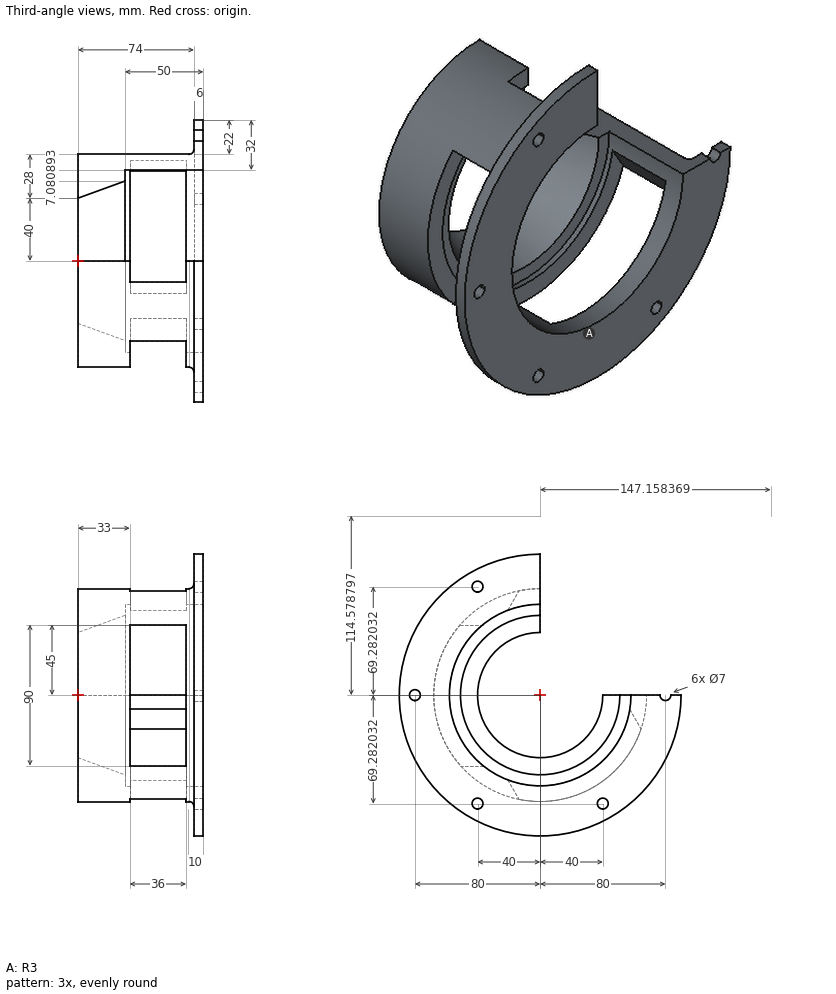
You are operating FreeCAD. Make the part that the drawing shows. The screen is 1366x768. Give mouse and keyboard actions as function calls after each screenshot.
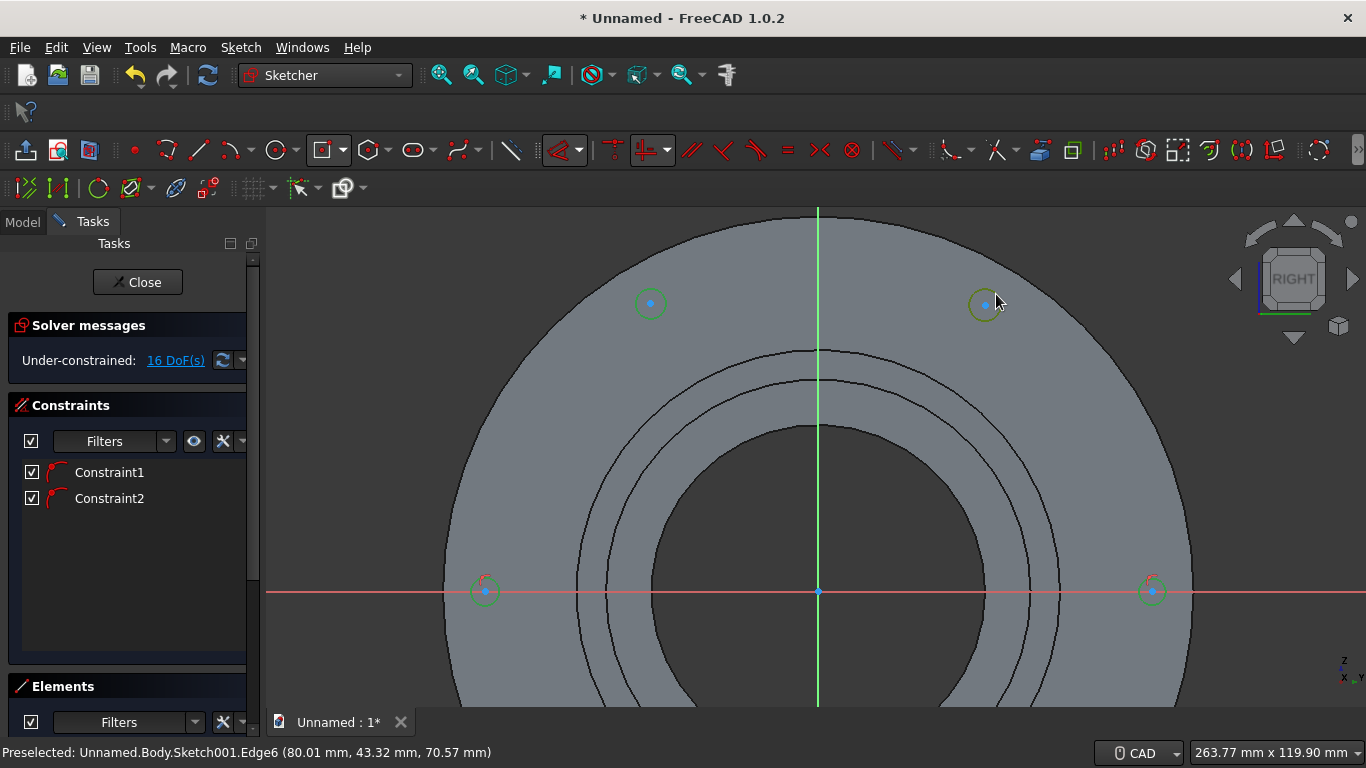
click(788, 150)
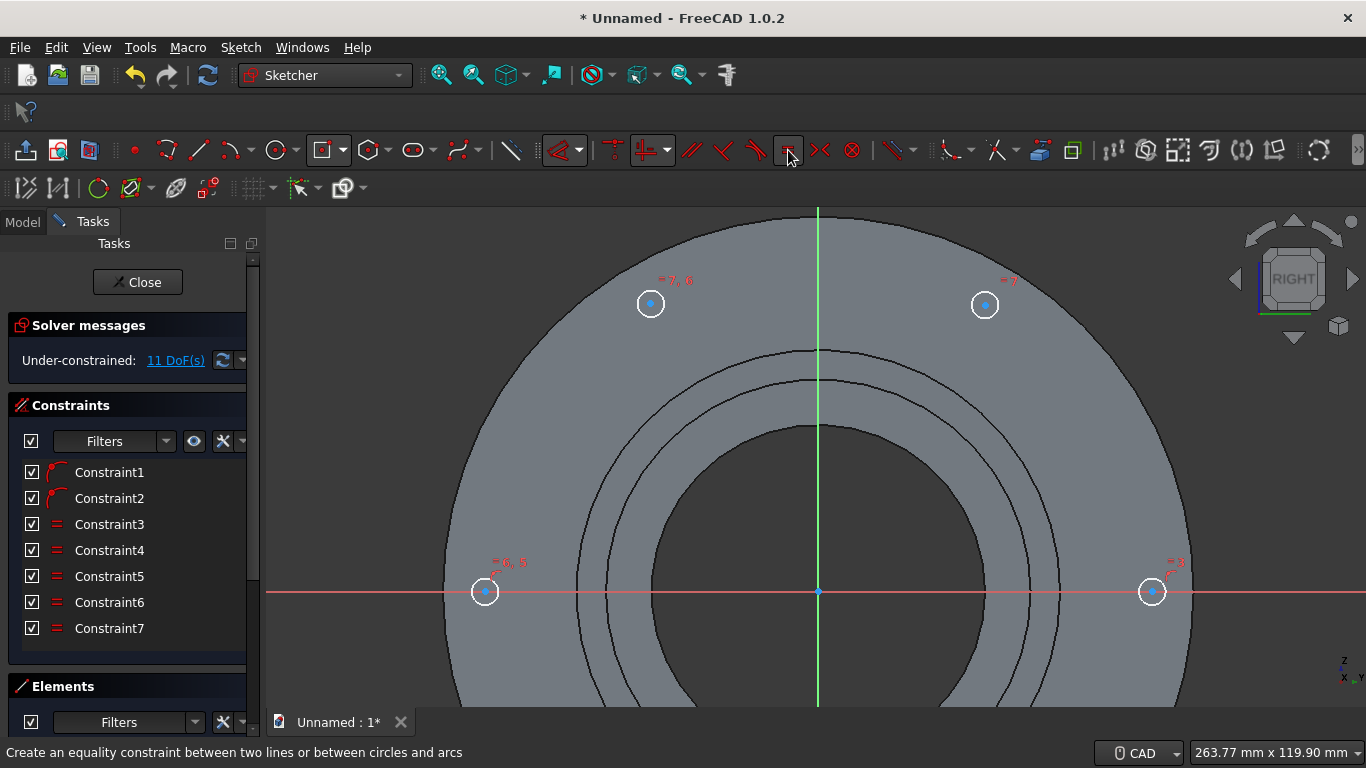
scroll(1162, 582, up, 2)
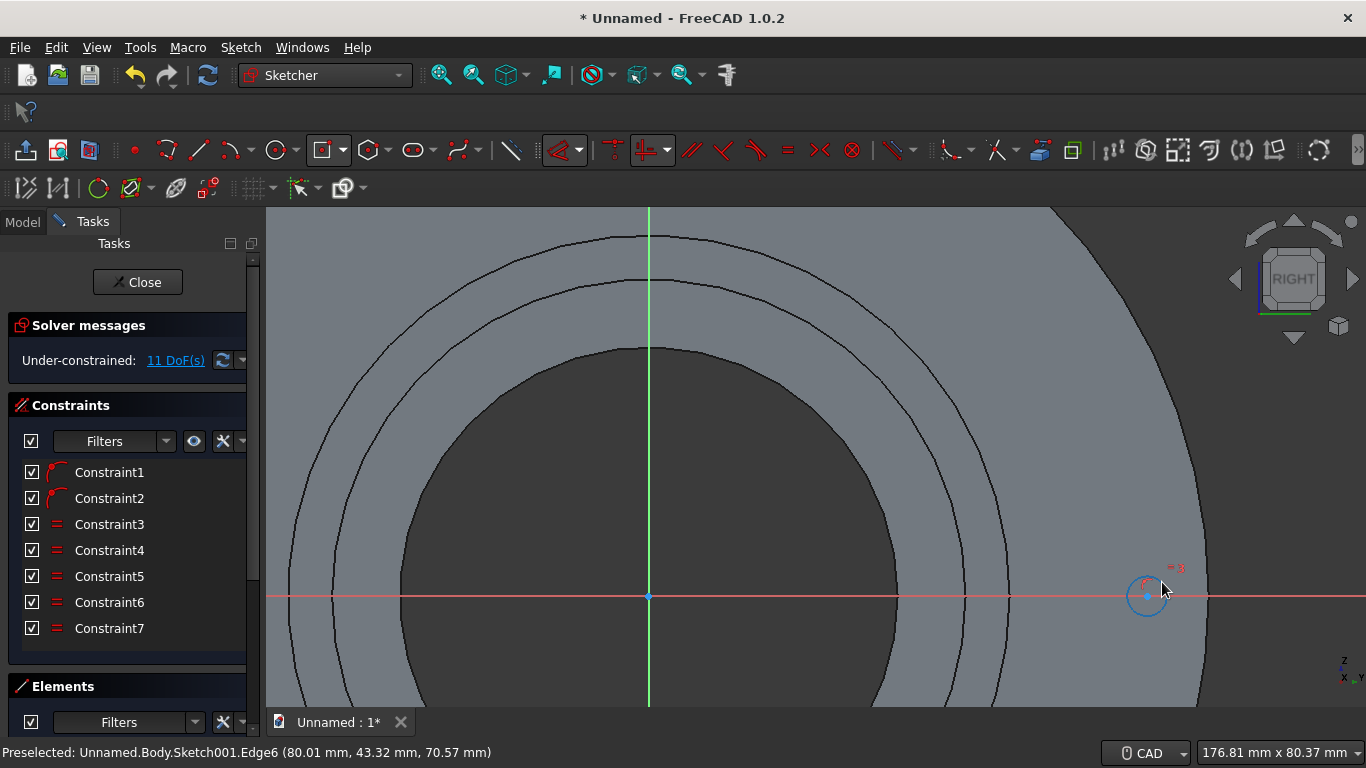
click(1161, 582)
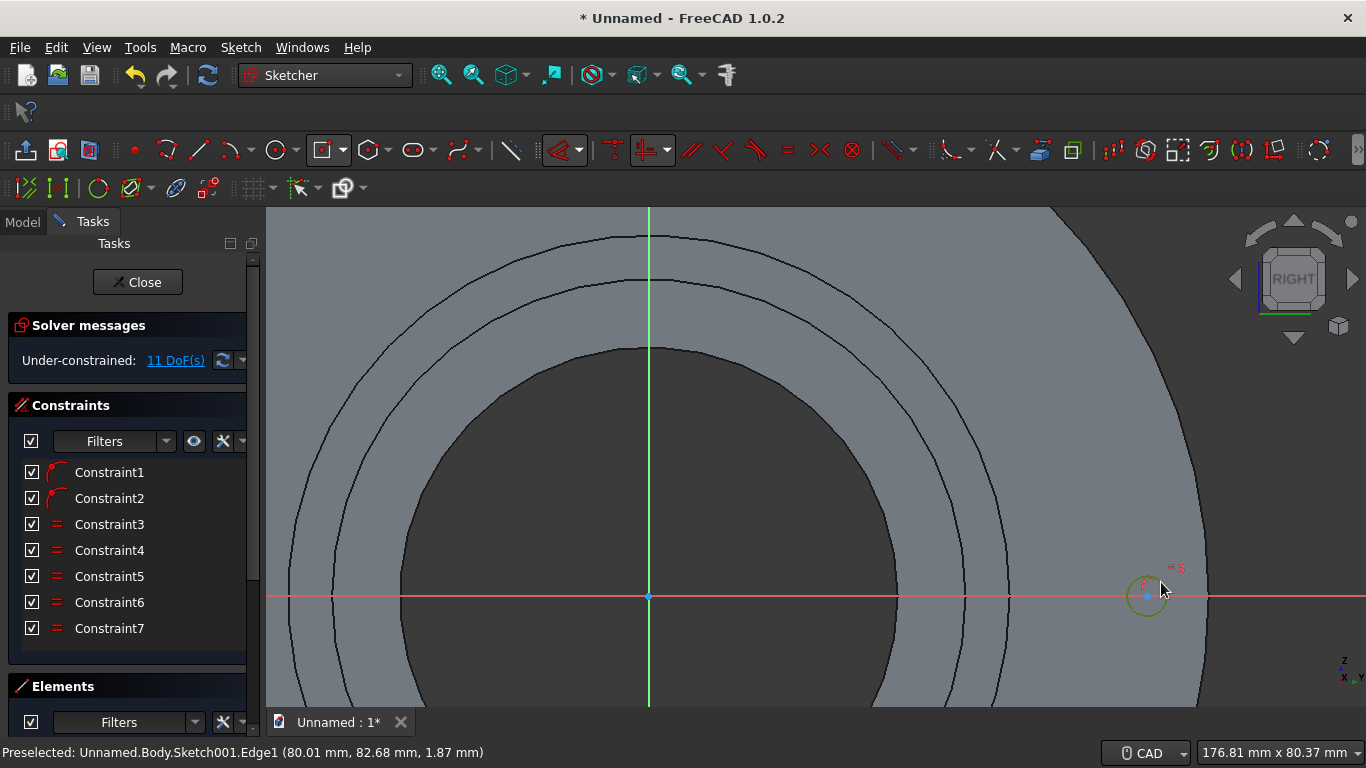
key(k)
key(o)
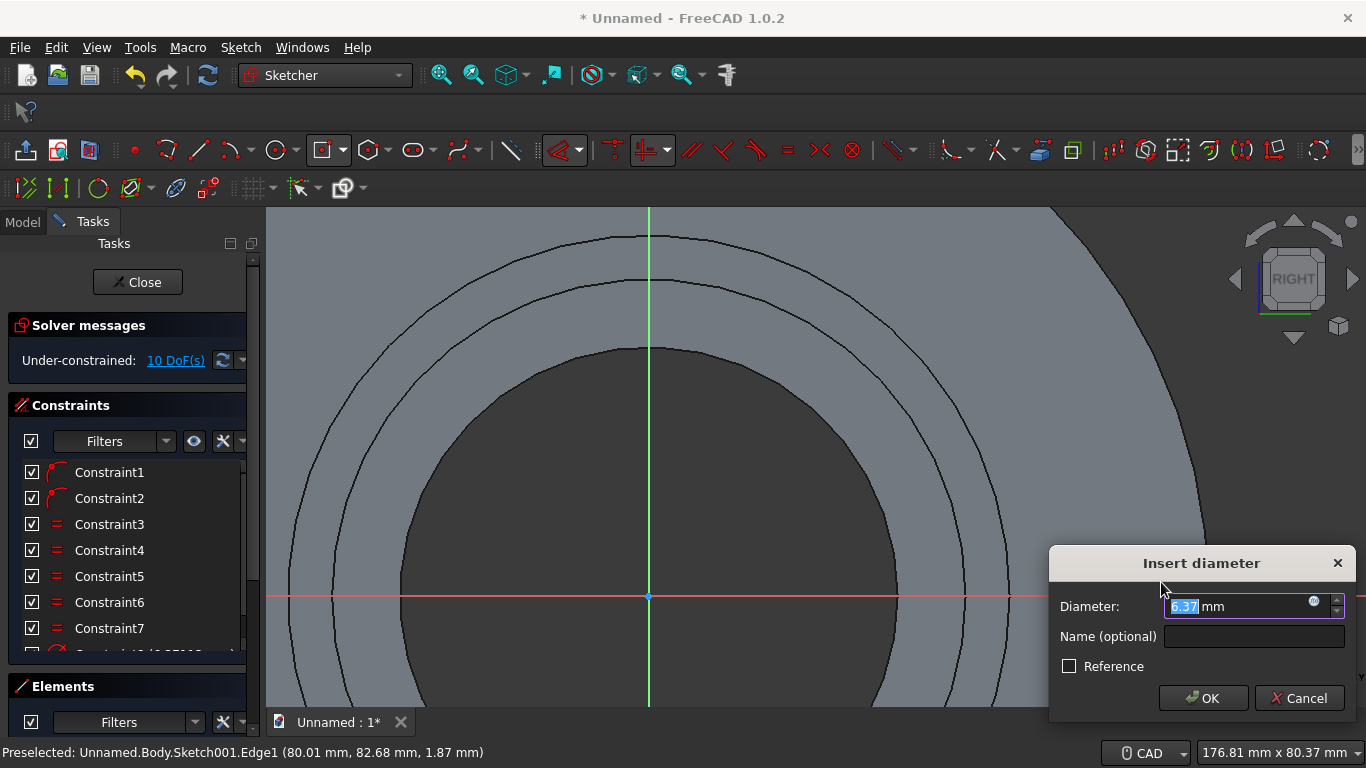
text(7)
key(Return)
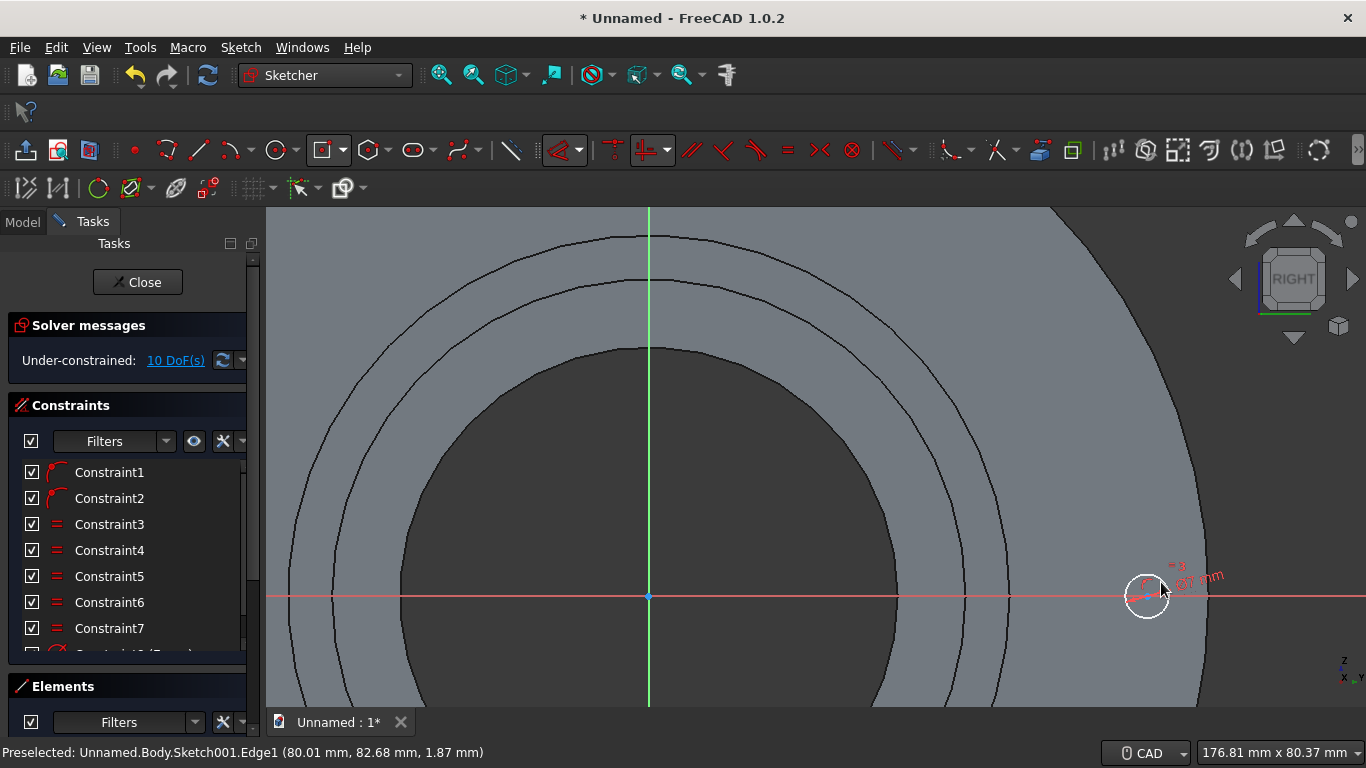
click(1147, 596)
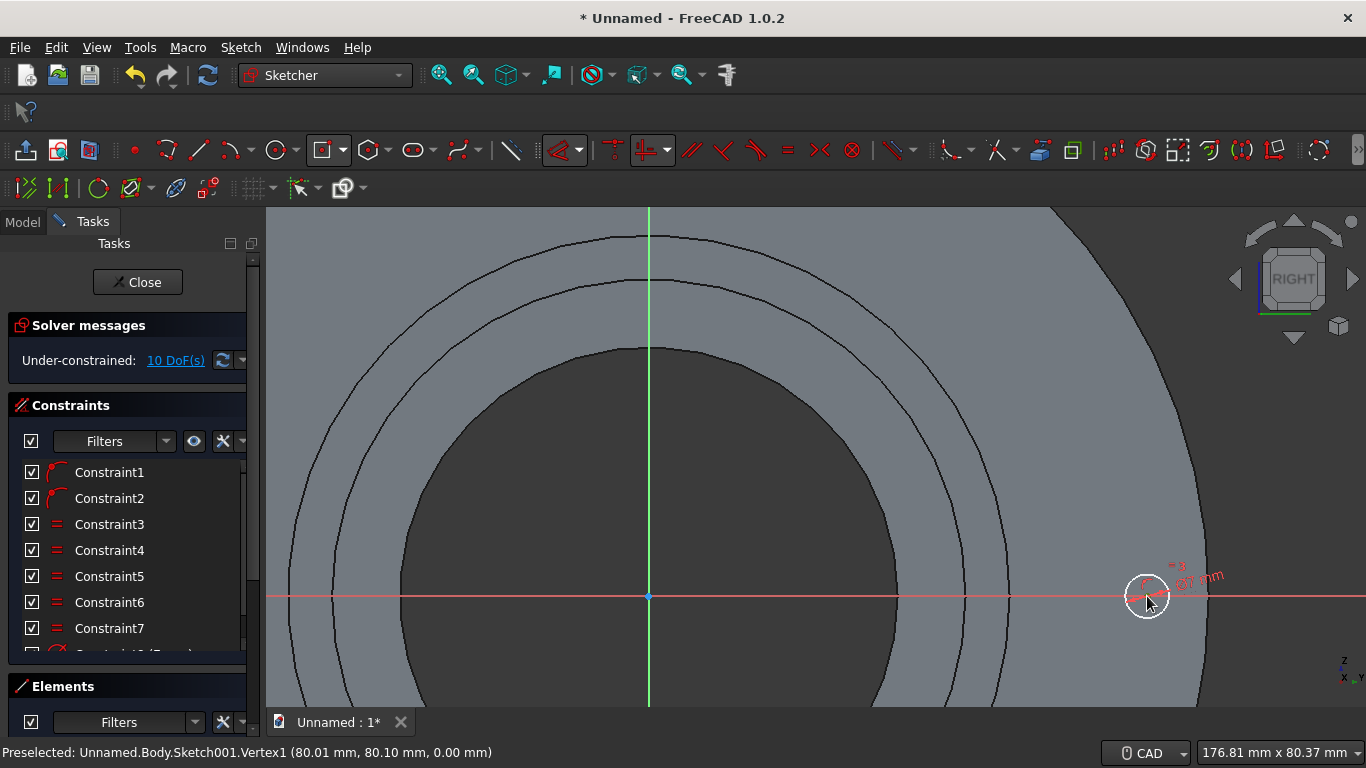
key(l)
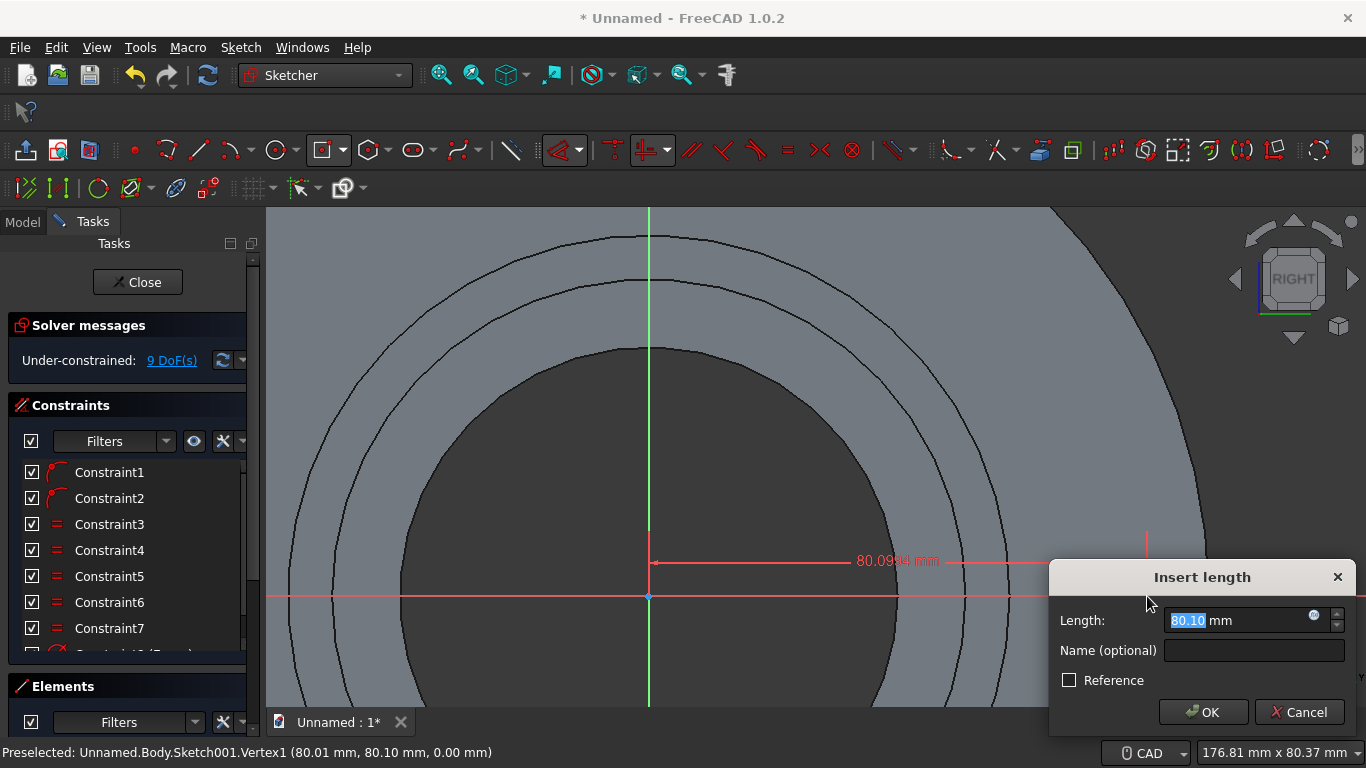
text(80)
key(Return)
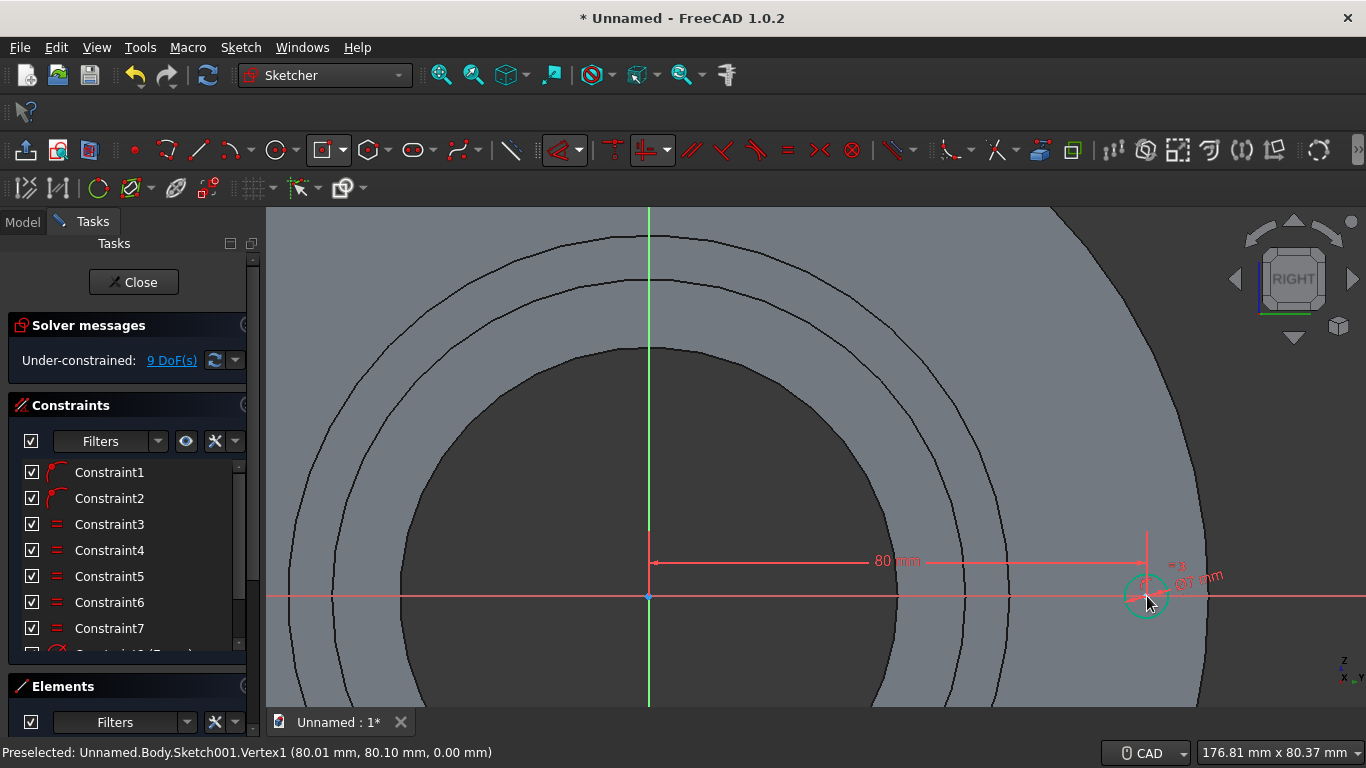
scroll(805, 376, down, 5)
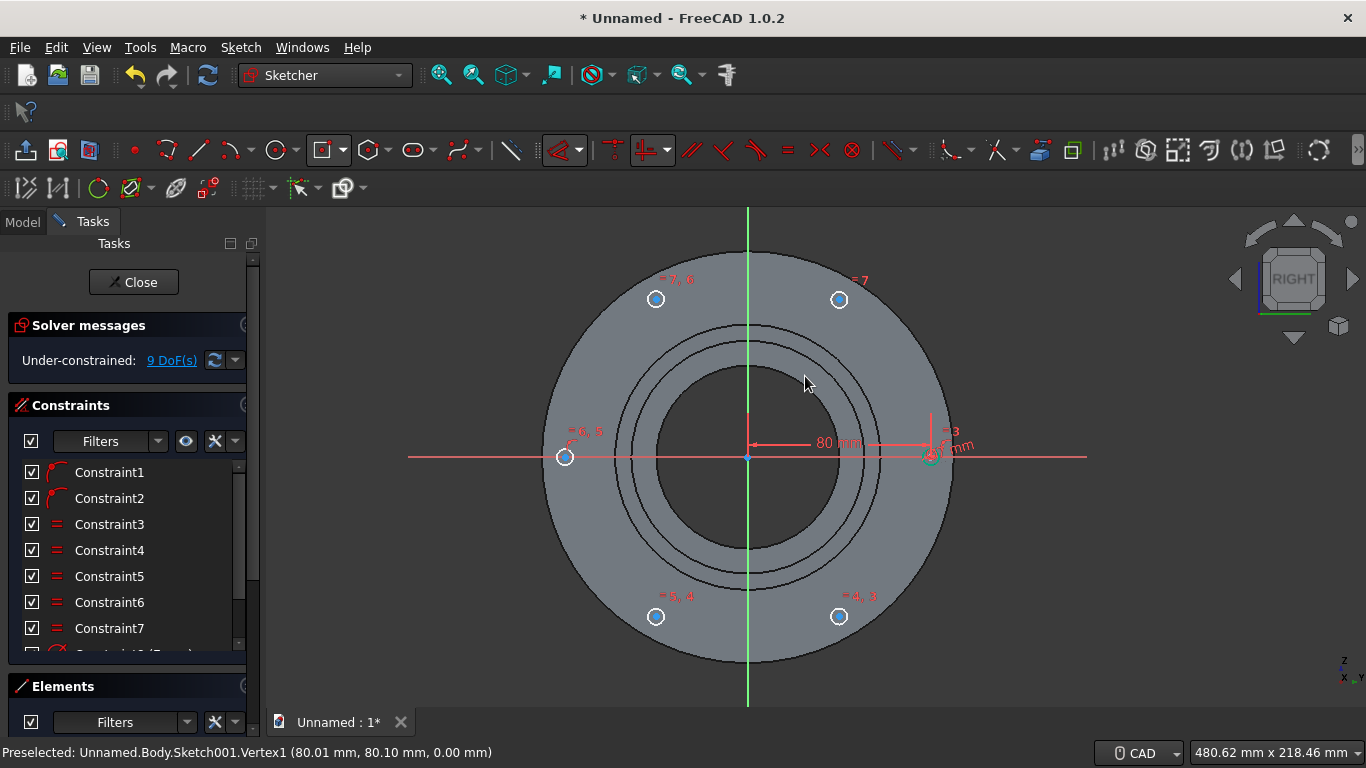
click(839, 616)